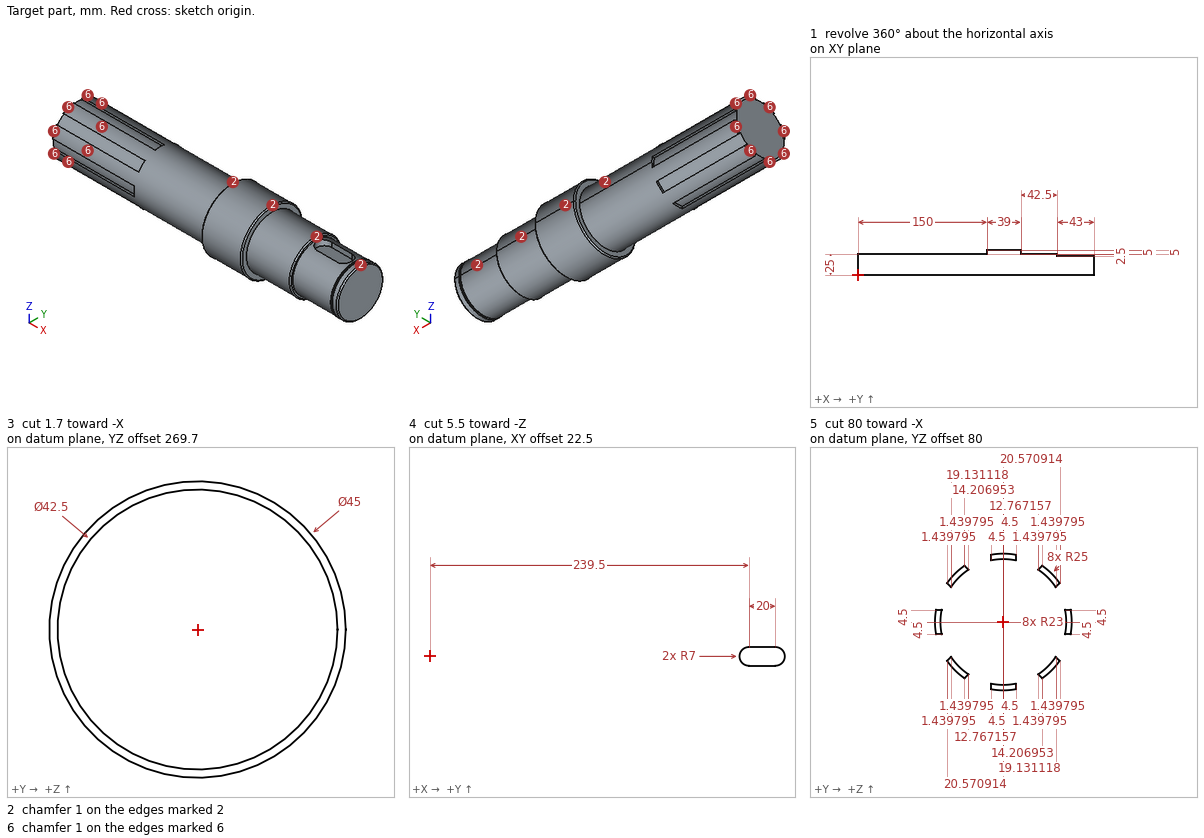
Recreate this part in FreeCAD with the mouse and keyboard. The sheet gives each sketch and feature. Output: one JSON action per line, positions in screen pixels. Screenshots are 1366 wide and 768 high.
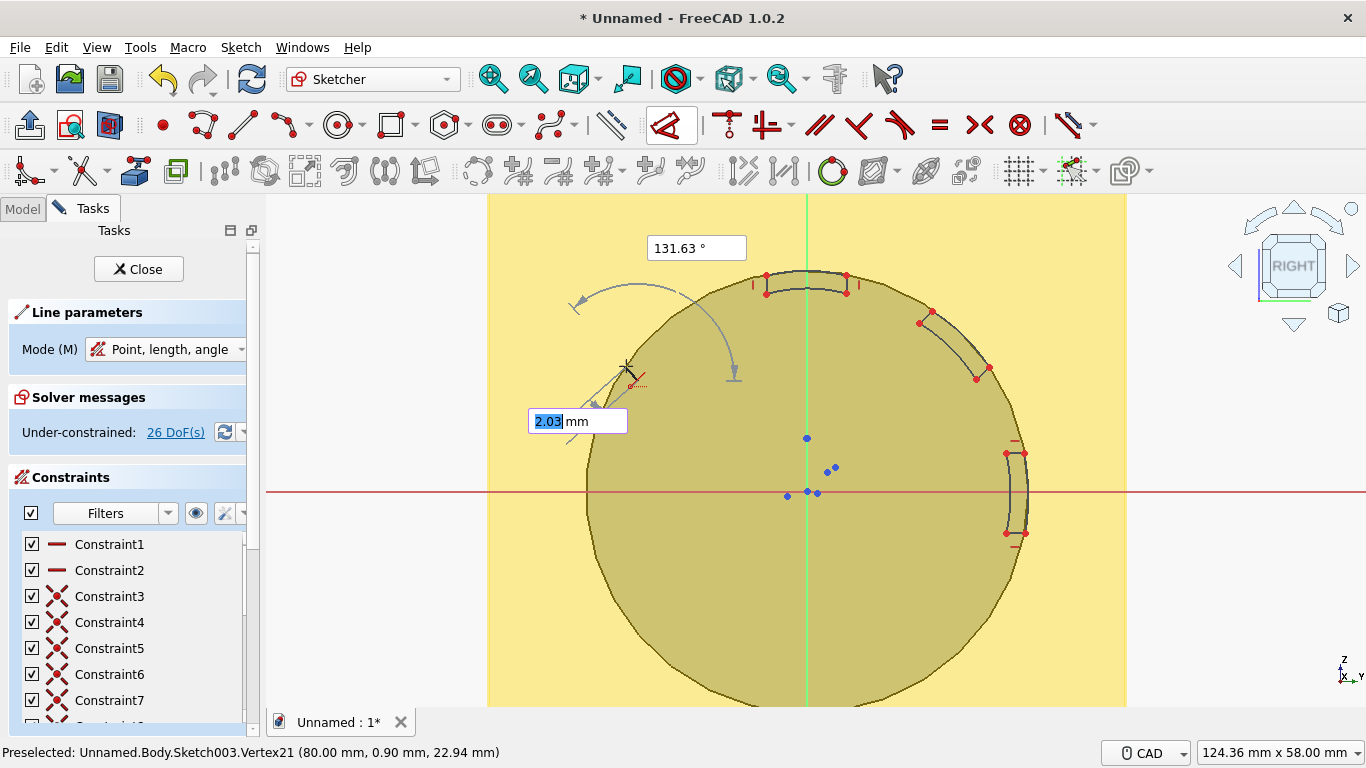
{"action": "left_click", "coordinate": [625, 366]}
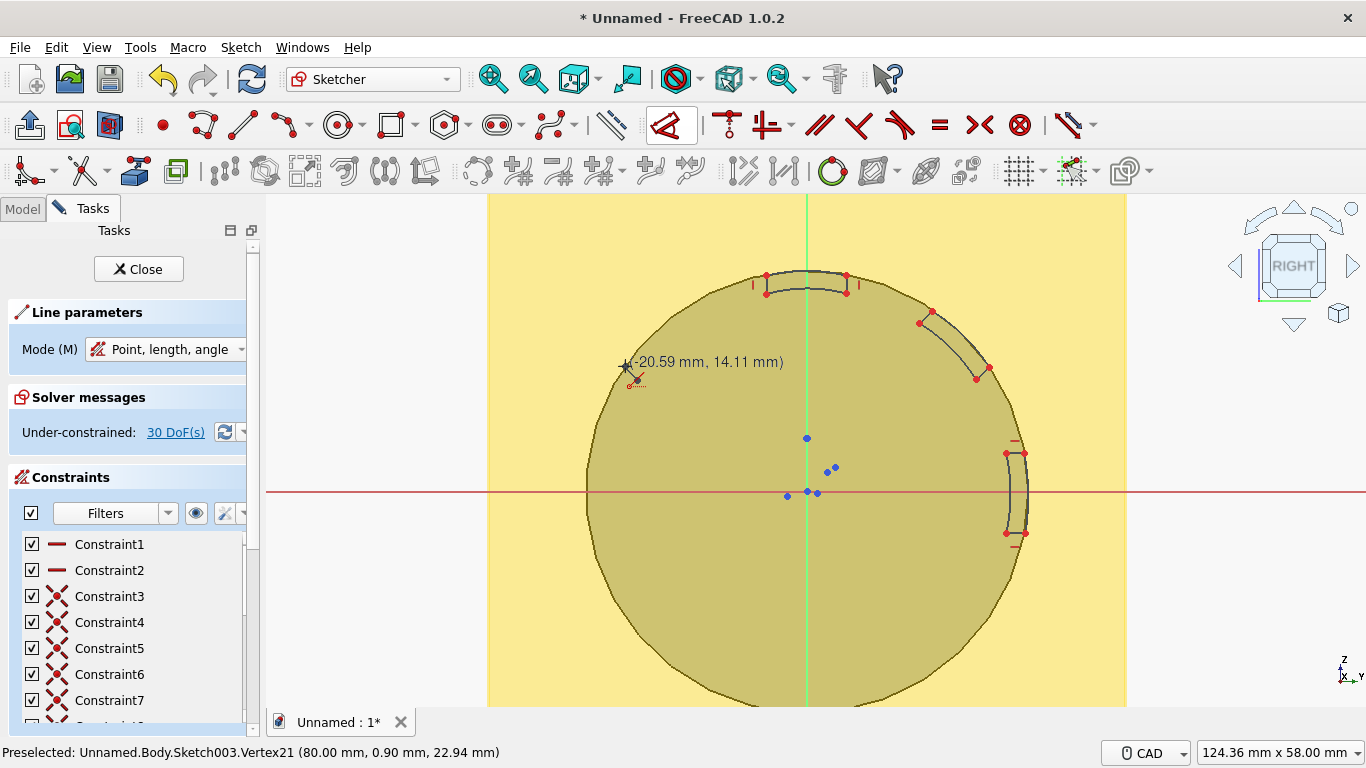
{"action": "left_click", "coordinate": [681, 310]}
{"action": "left_click", "coordinate": [694, 323]}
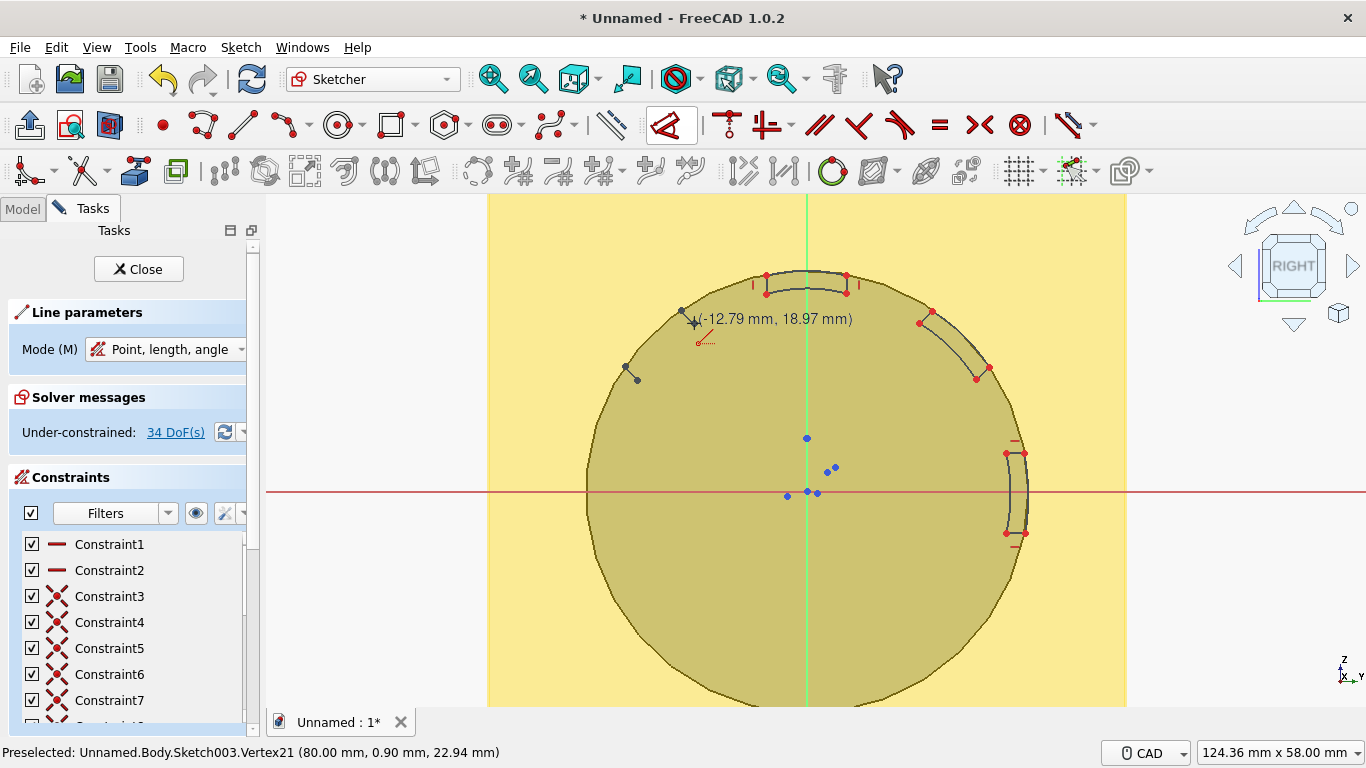
{"action": "left_click", "coordinate": [284, 126]}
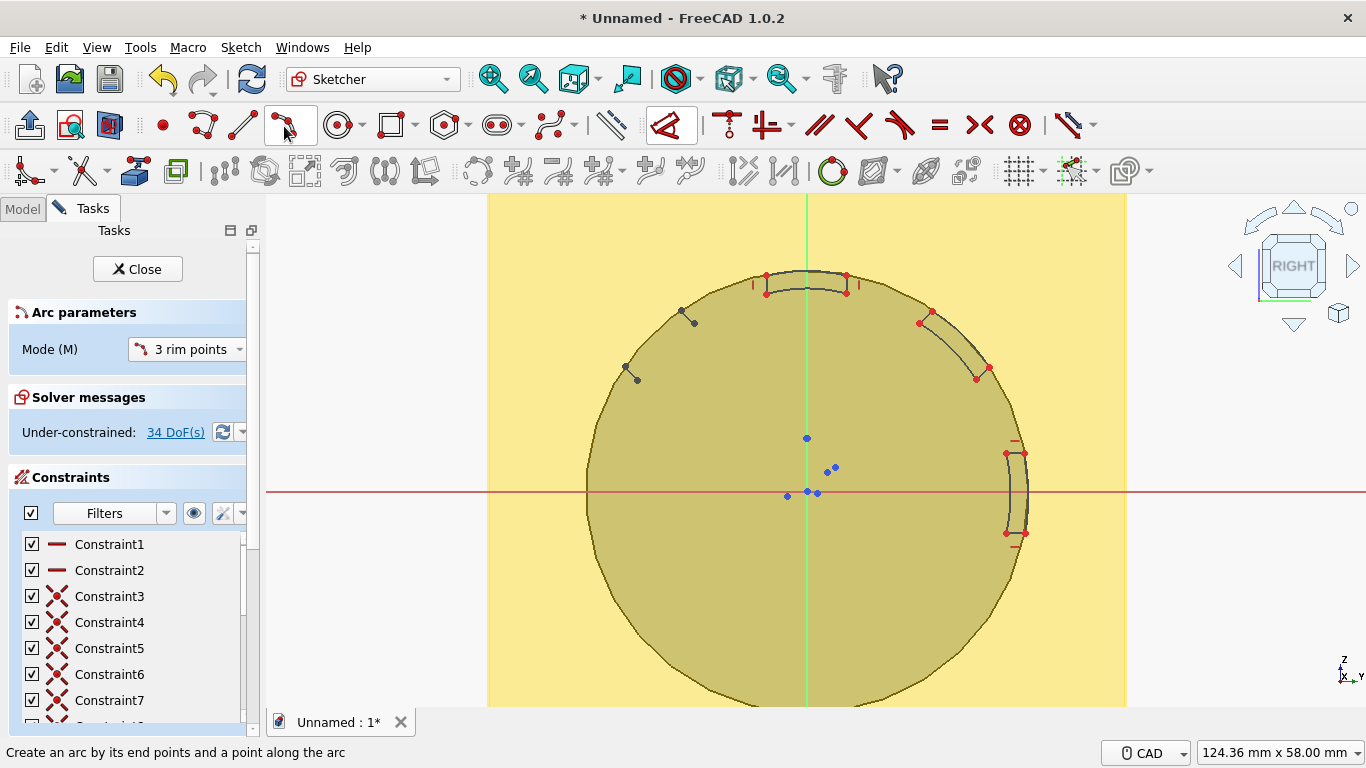
{"action": "scroll", "coordinate": [625, 366], "scroll_direction": "up", "scroll_amount": 3}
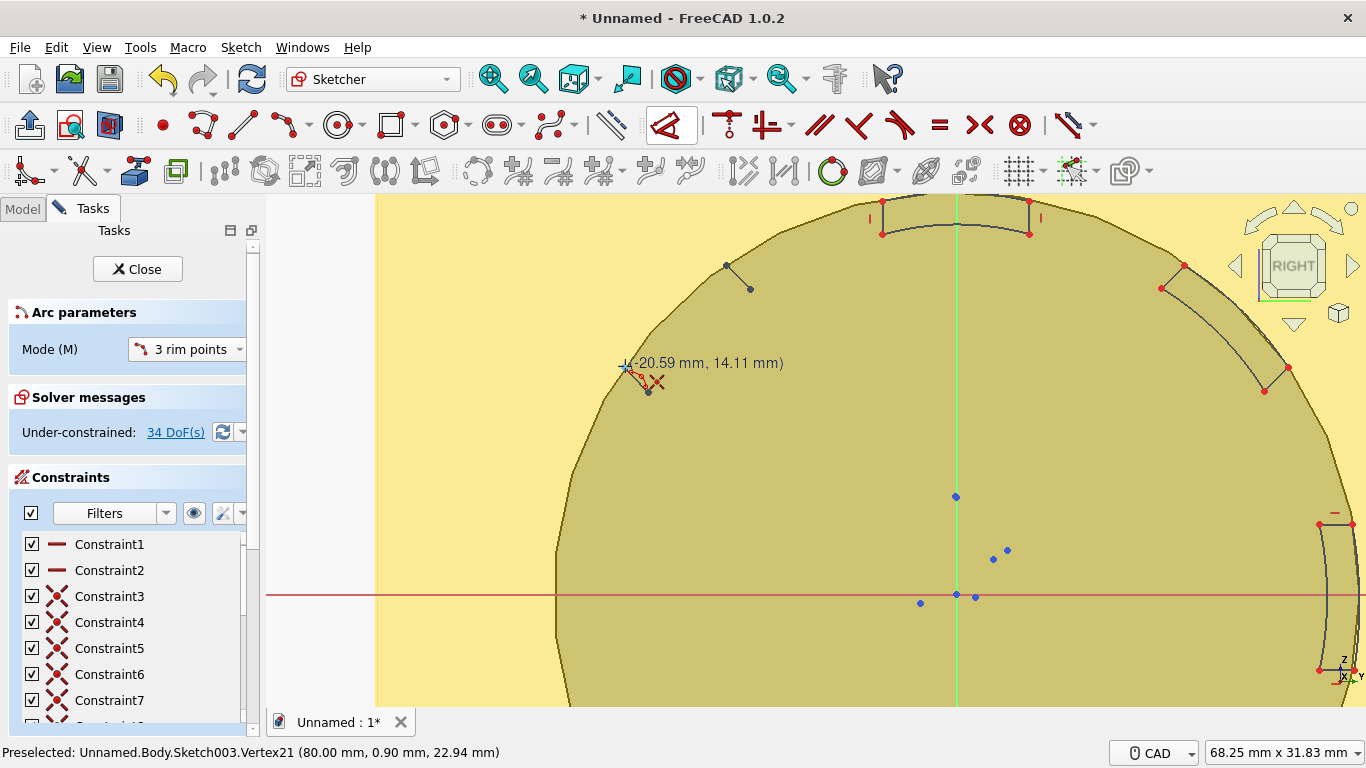
{"action": "left_click", "coordinate": [625, 368]}
{"action": "left_click", "coordinate": [727, 266]}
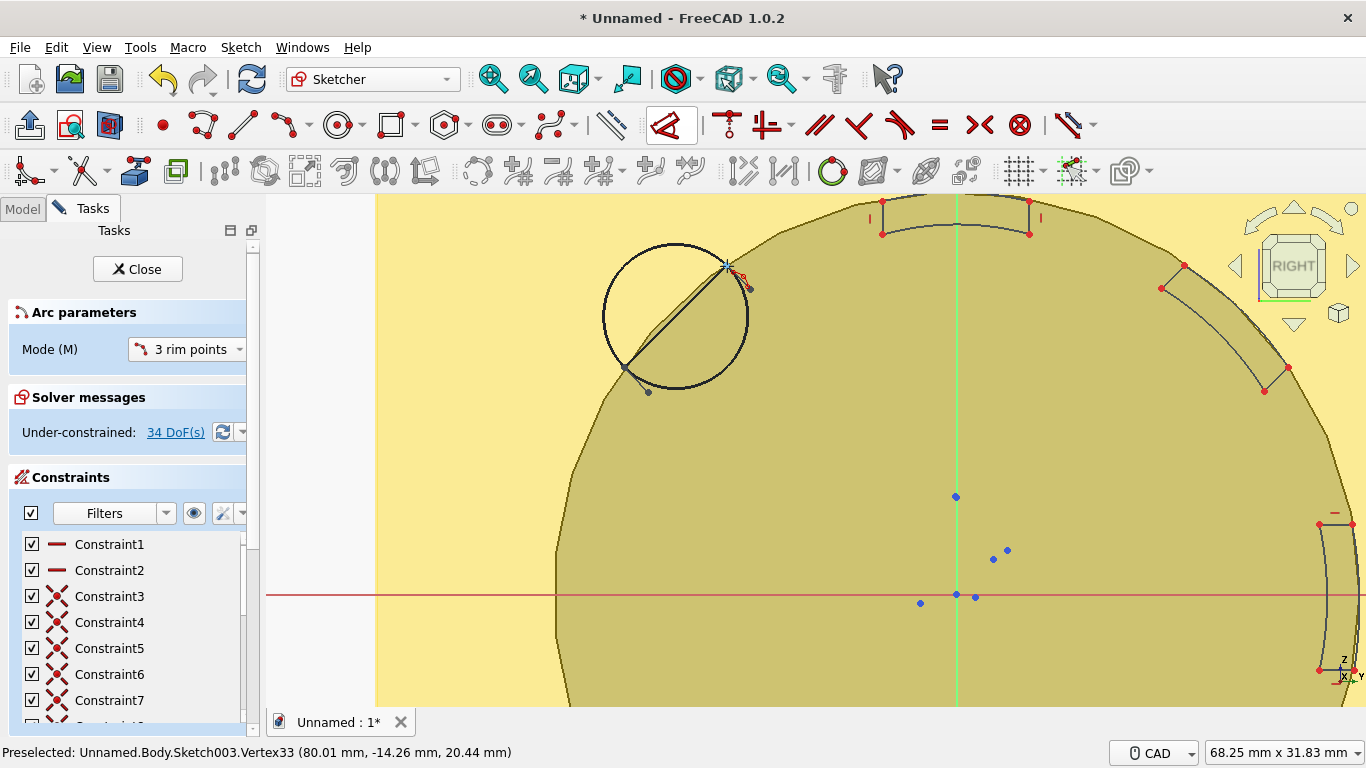
{"action": "scroll", "coordinate": [672, 310], "scroll_direction": "up", "scroll_amount": 5}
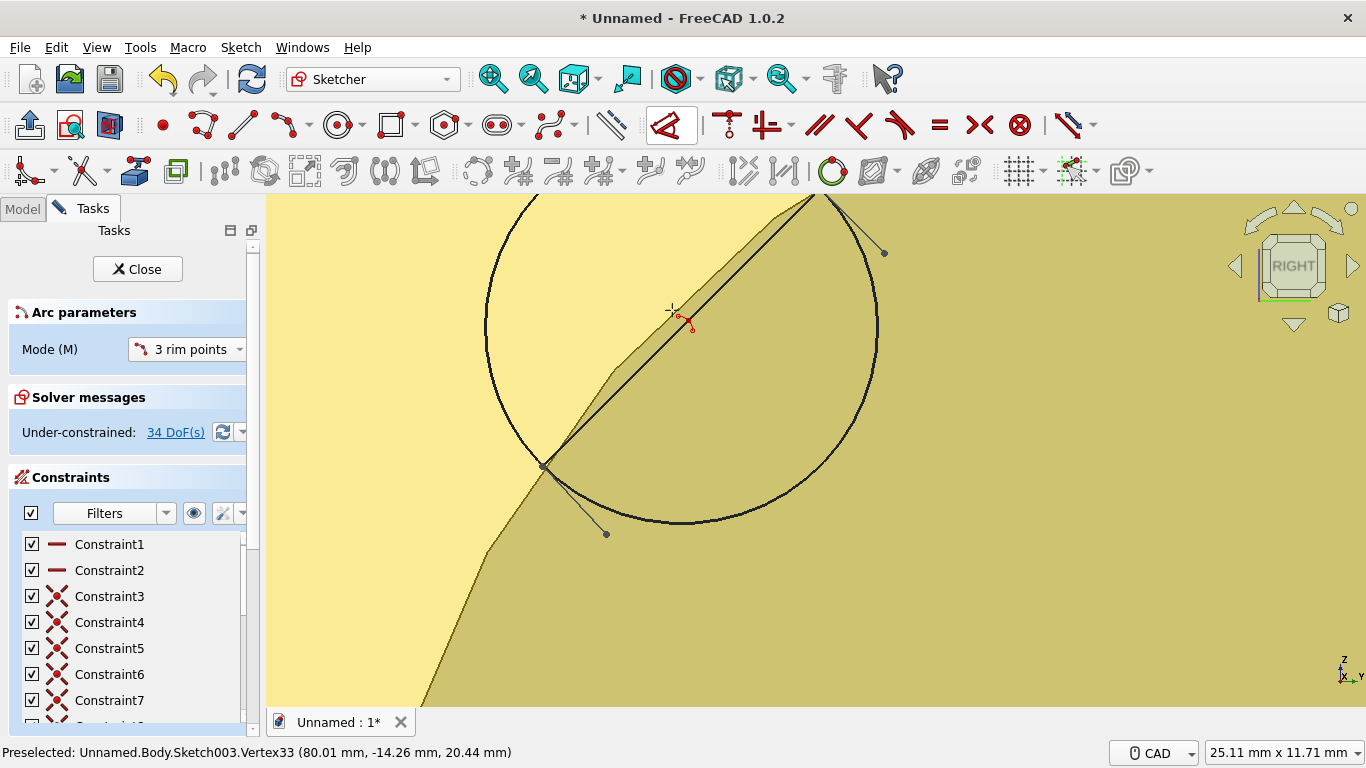
{"action": "left_click", "coordinate": [671, 310]}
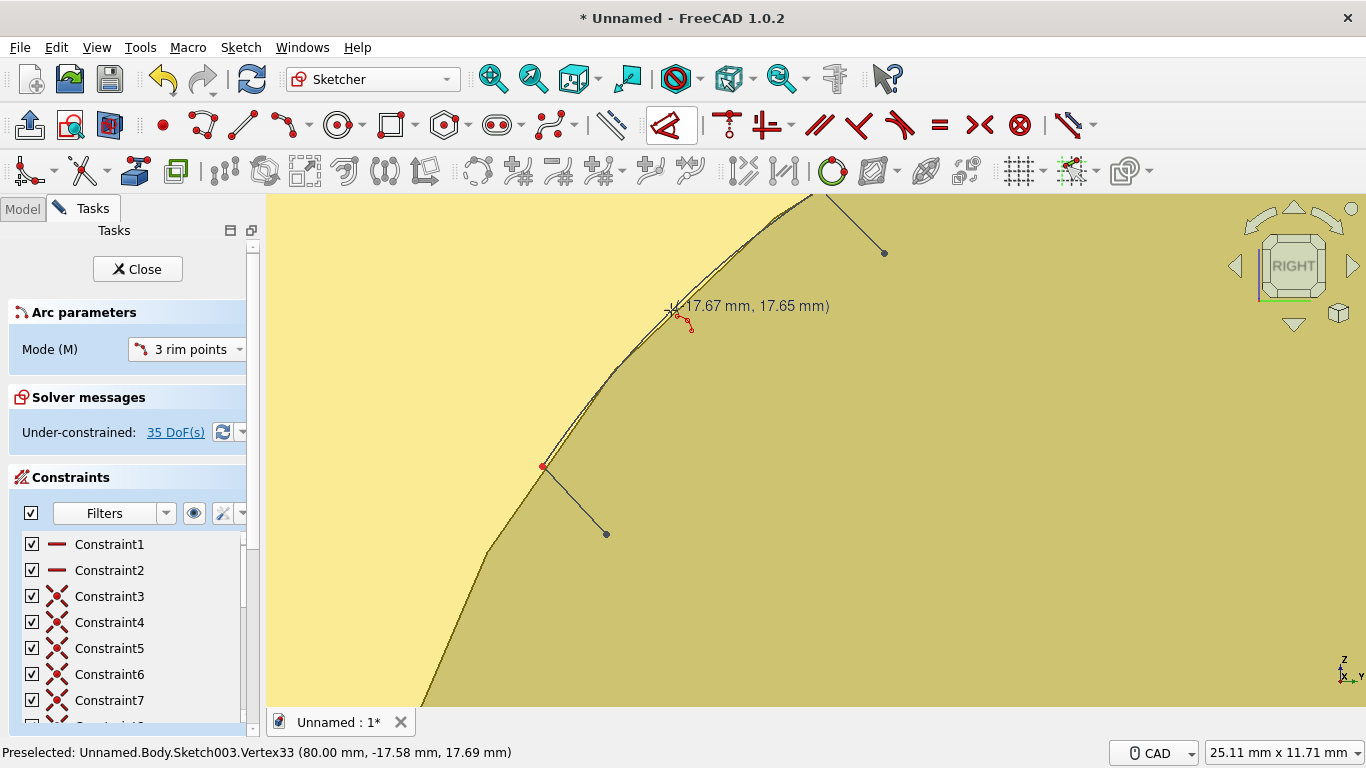
{"action": "left_click", "coordinate": [885, 253]}
{"action": "left_click", "coordinate": [606, 534]}
{"action": "left_click", "coordinate": [733, 372]}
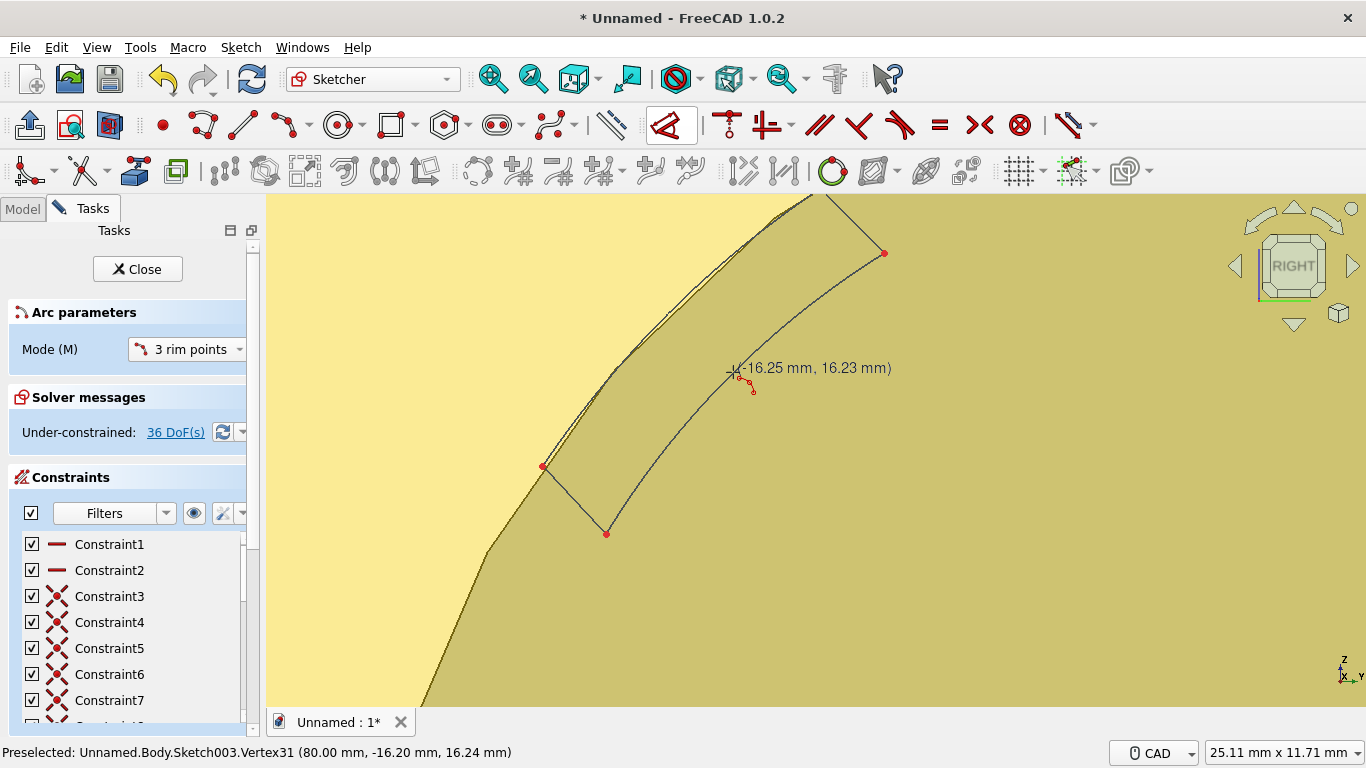
{"action": "left_click", "coordinate": [244, 126]}